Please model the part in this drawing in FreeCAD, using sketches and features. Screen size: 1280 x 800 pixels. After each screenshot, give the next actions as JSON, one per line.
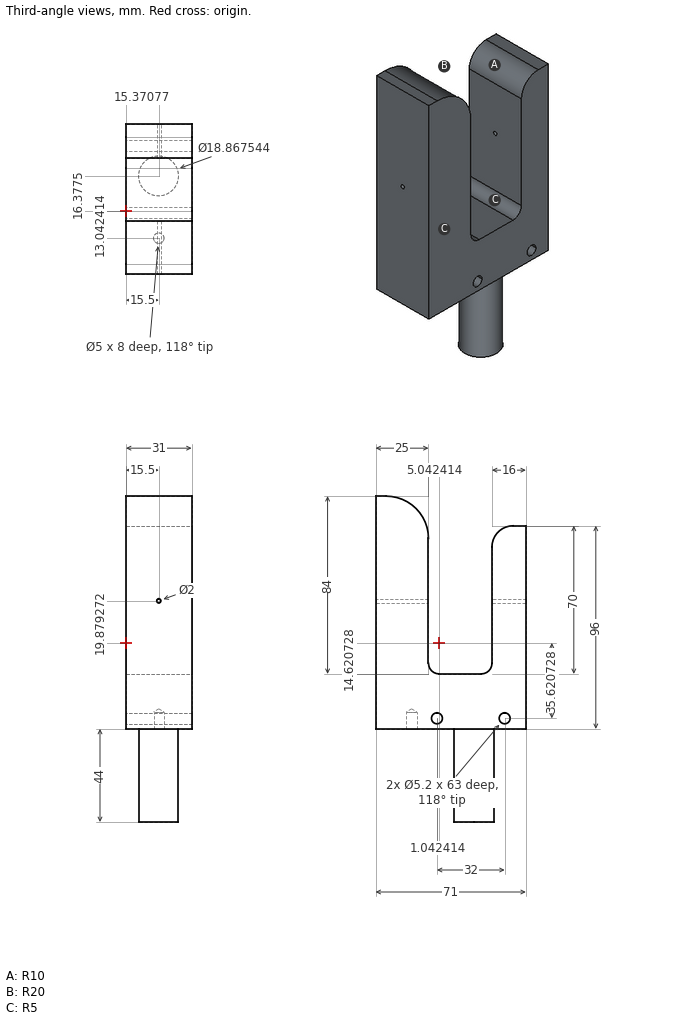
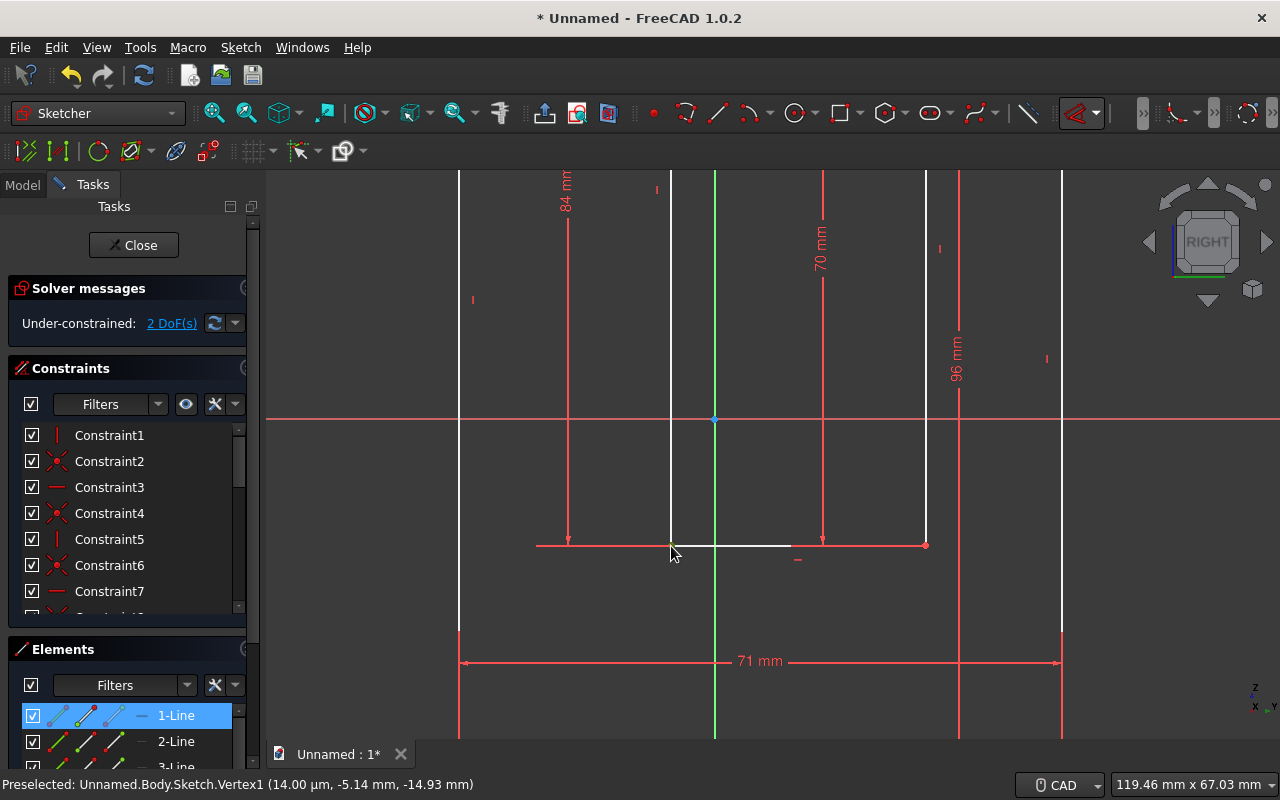
{"action": "left_click", "coordinate": [1098, 114]}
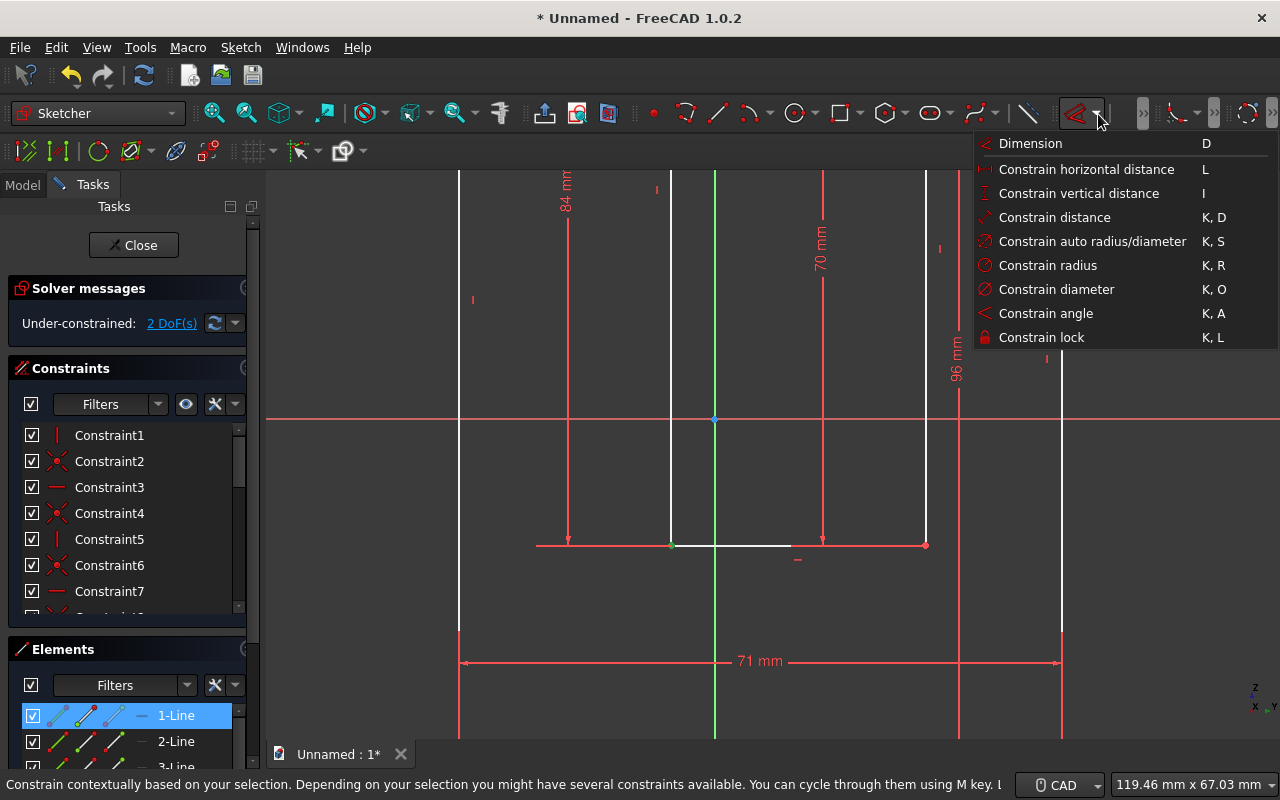
{"action": "left_click", "coordinate": [1126, 169]}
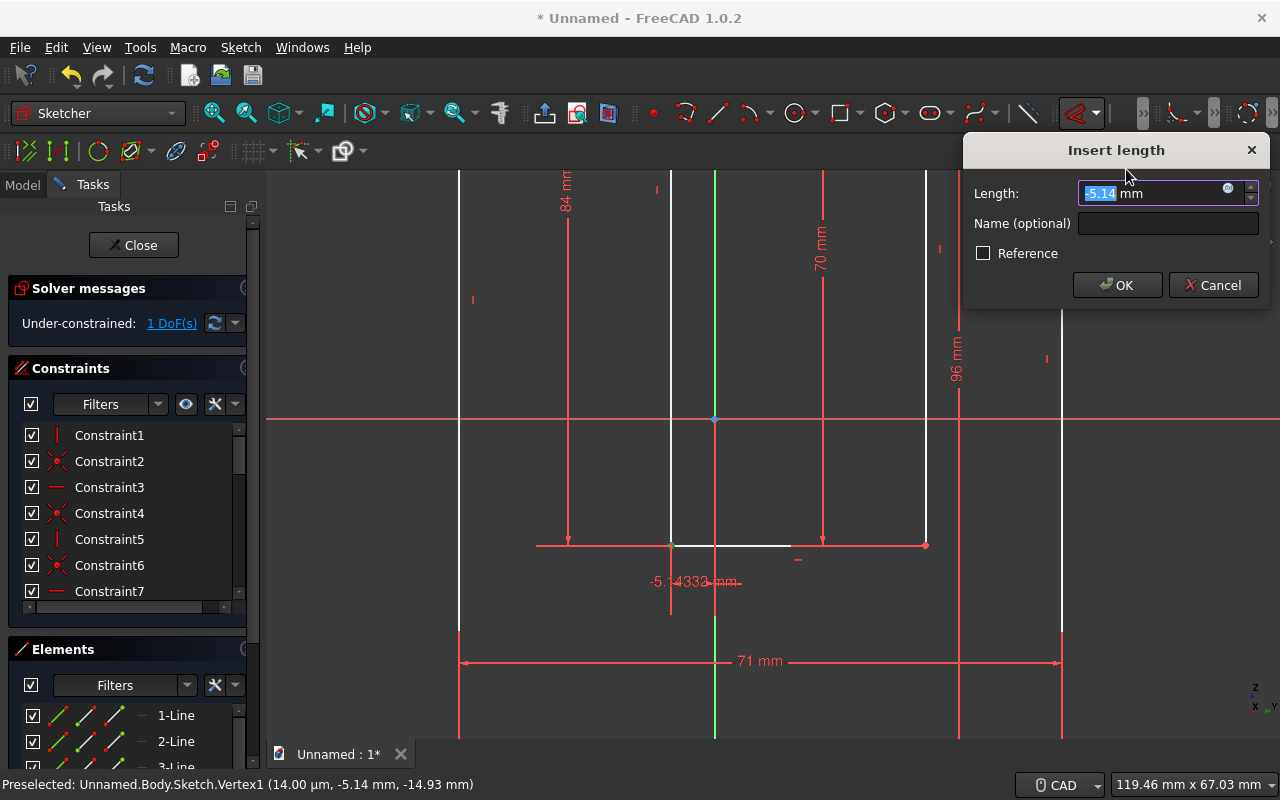
{"action": "type", "text": "-5.042414"}
{"action": "key", "text": "Return"}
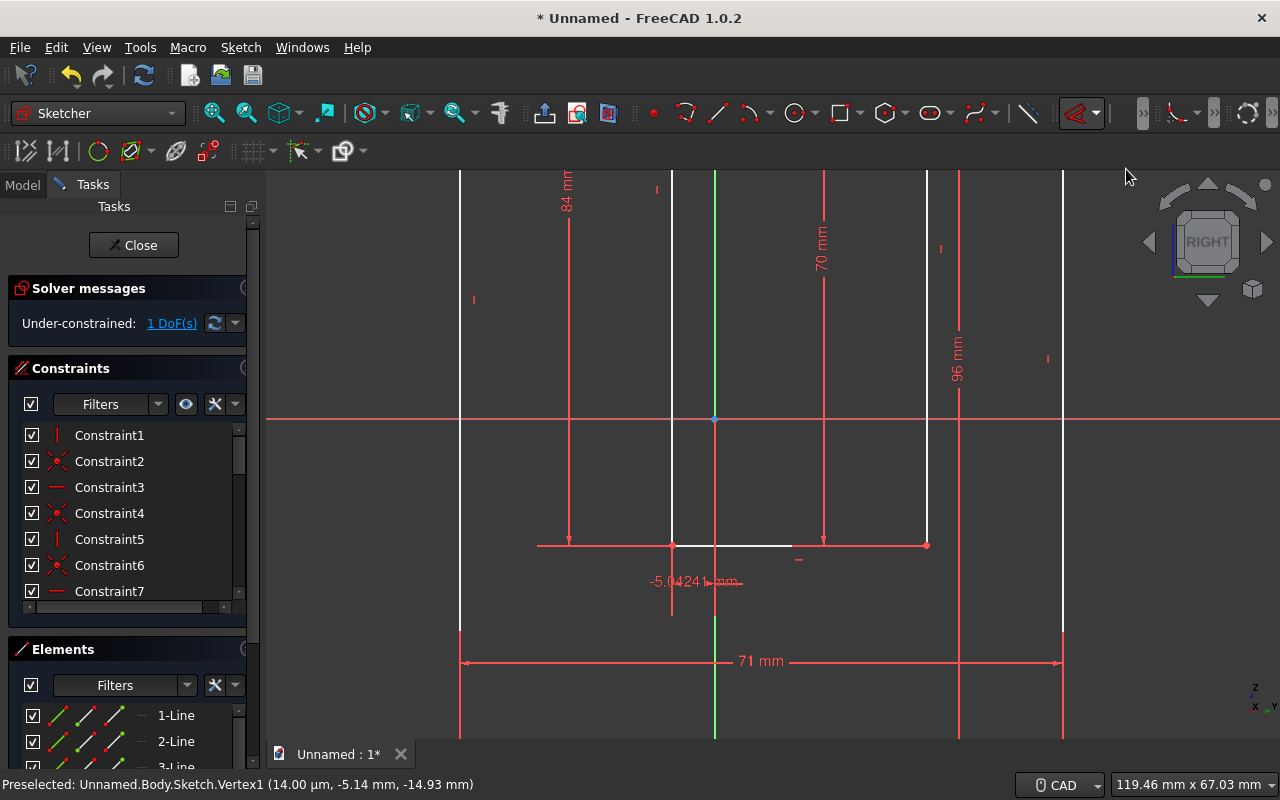
{"action": "left_click", "coordinate": [672, 546]}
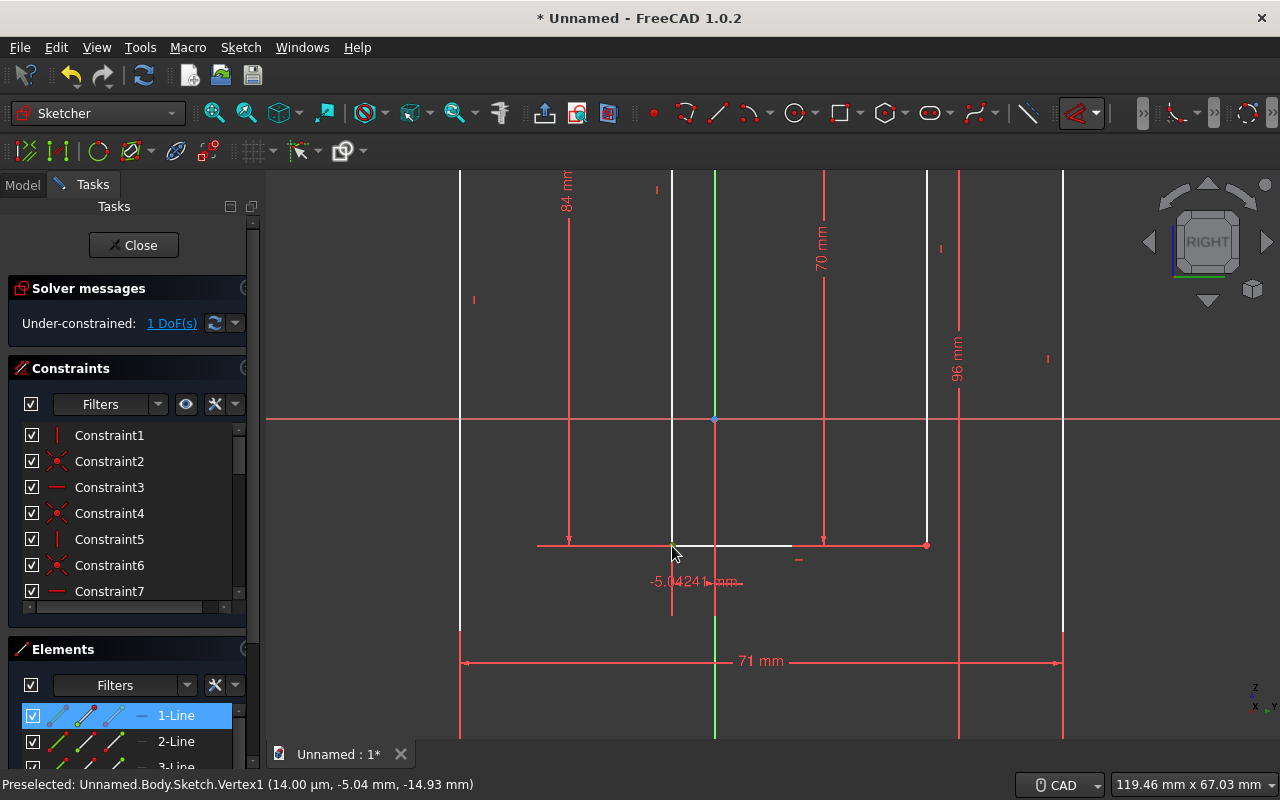
{"action": "left_click", "coordinate": [1098, 114]}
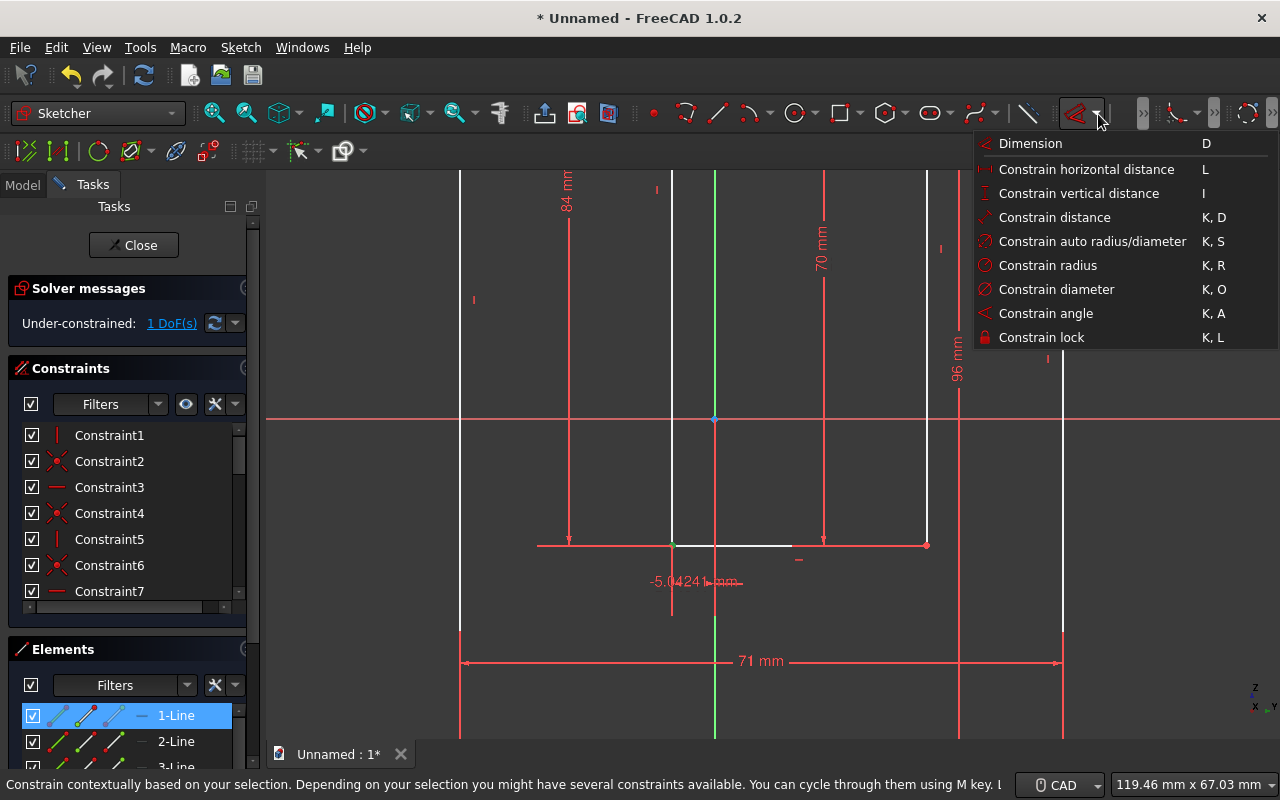
{"action": "left_click", "coordinate": [1126, 193]}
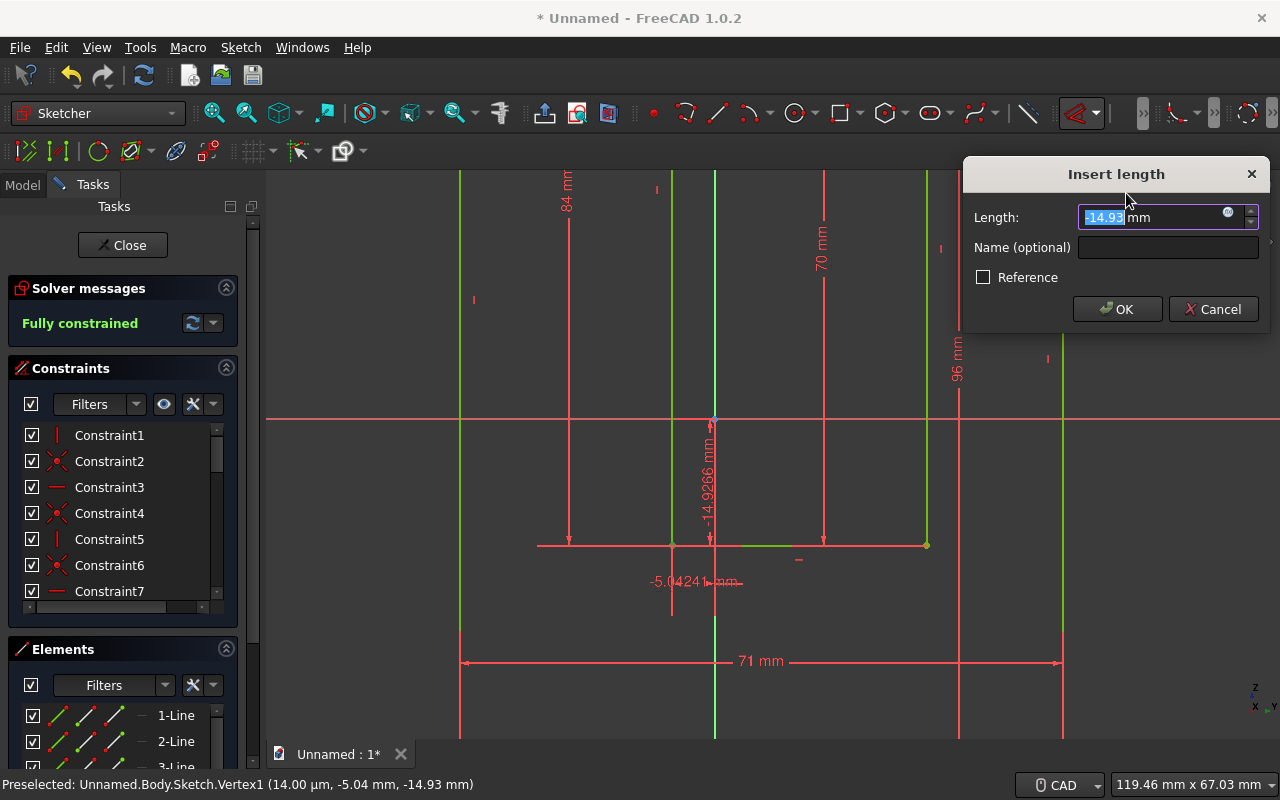
{"action": "type", "text": "-14.620728"}
{"action": "key", "text": "Return"}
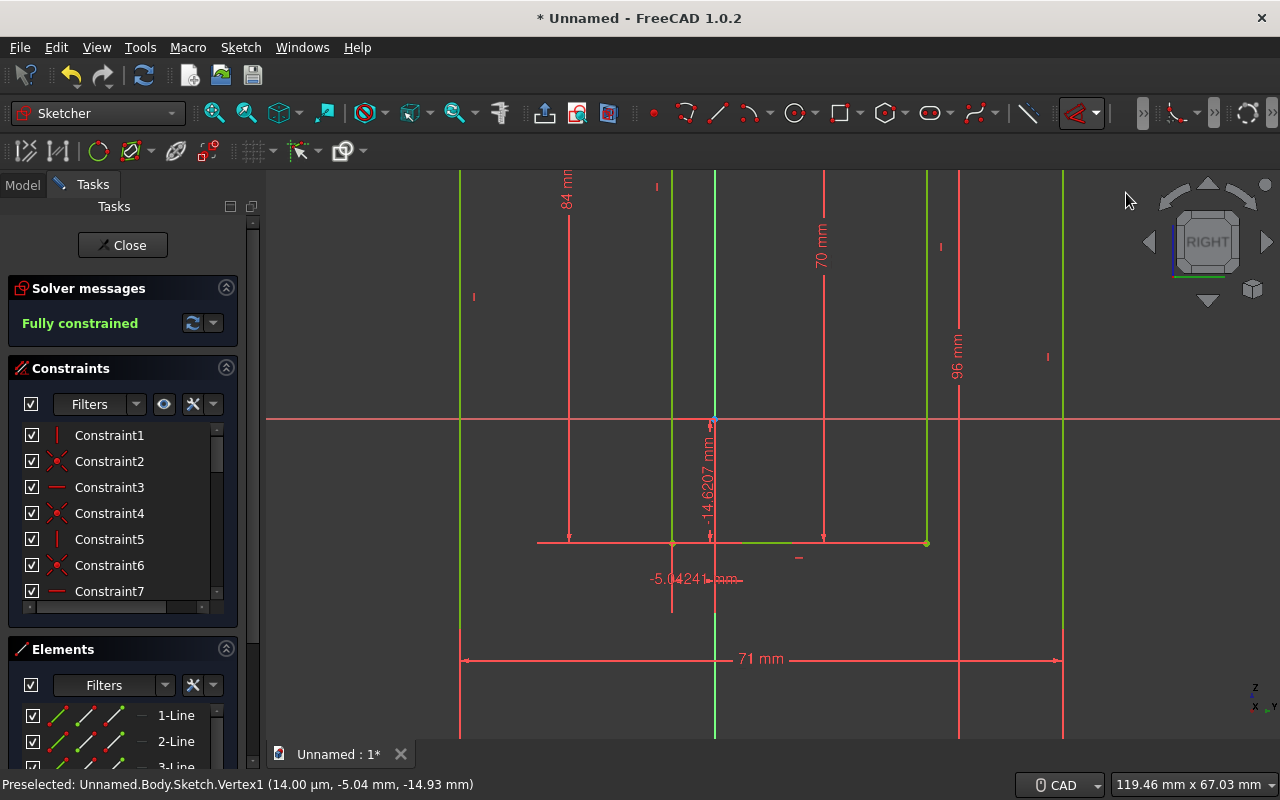
{"action": "left_click", "coordinate": [123, 245]}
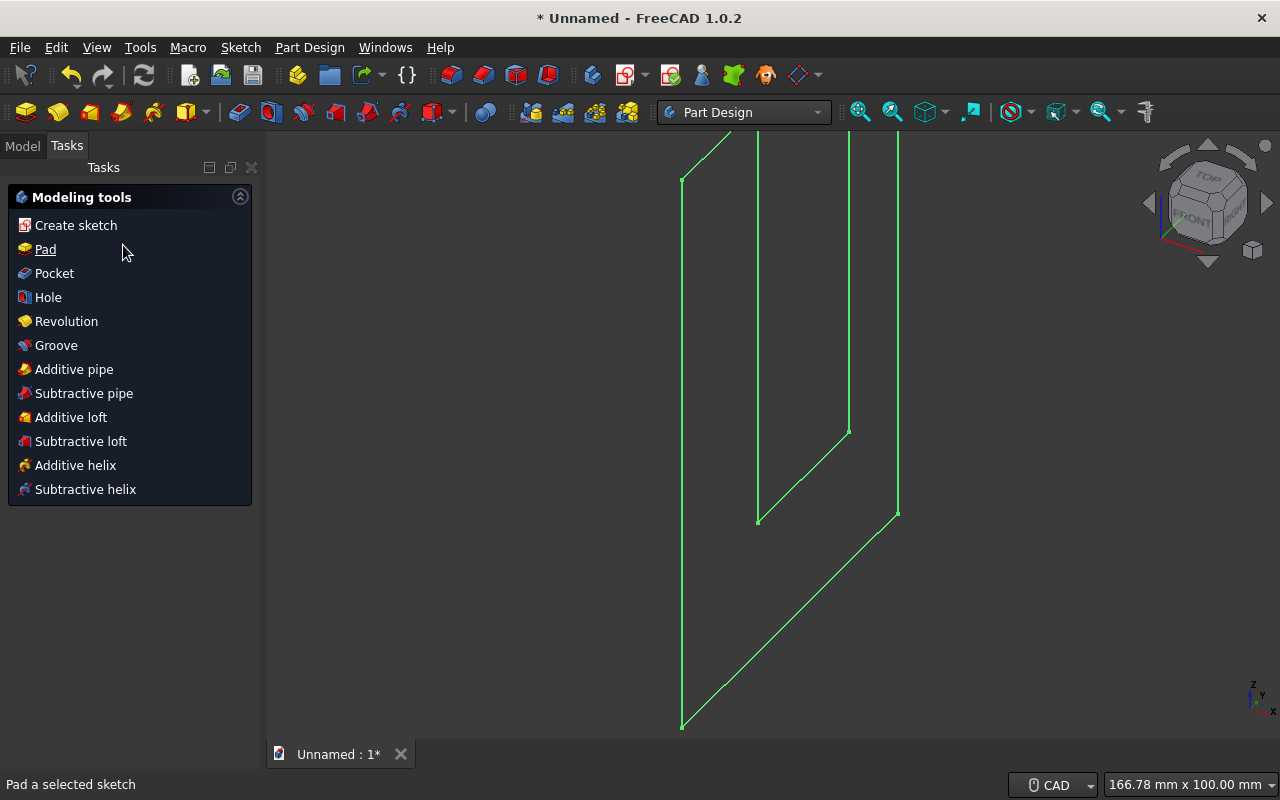
{"action": "left_click", "coordinate": [26, 112]}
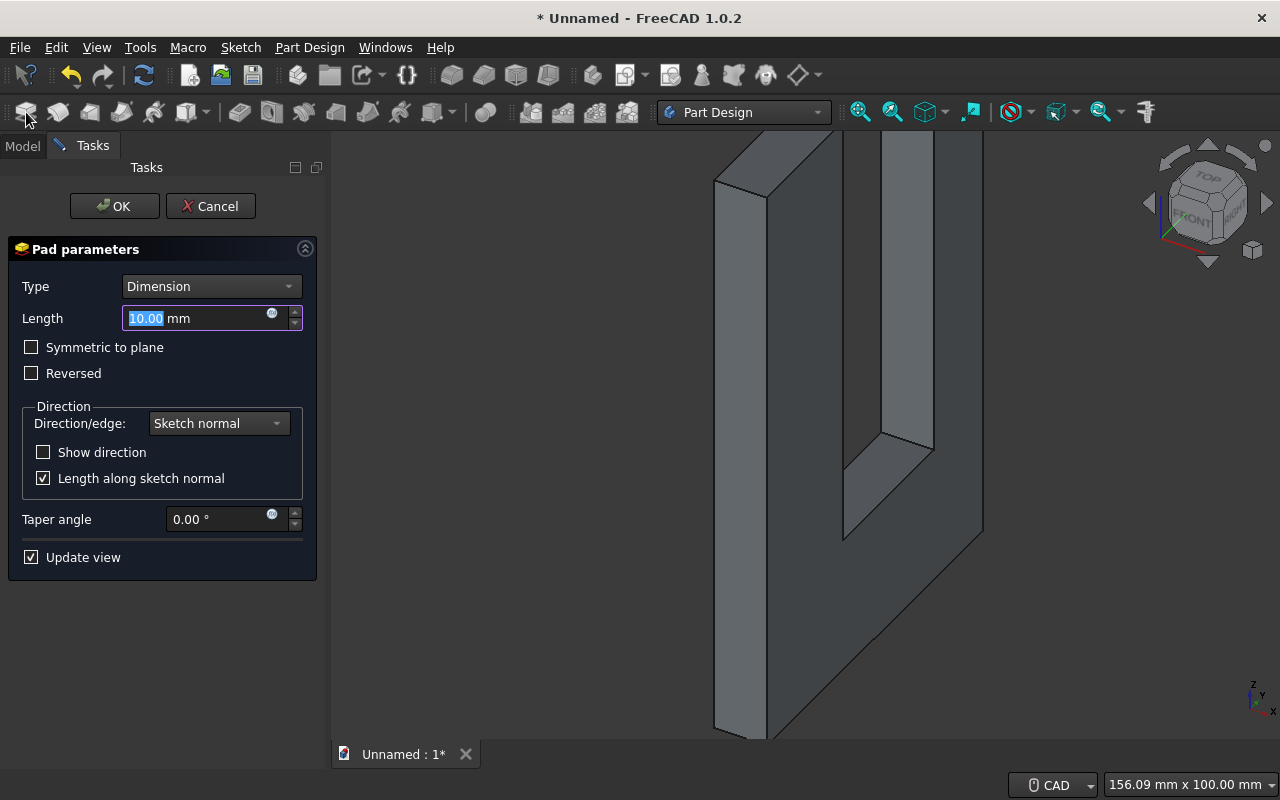
{"action": "type", "text": "31"}
{"action": "key", "text": "Tab"}